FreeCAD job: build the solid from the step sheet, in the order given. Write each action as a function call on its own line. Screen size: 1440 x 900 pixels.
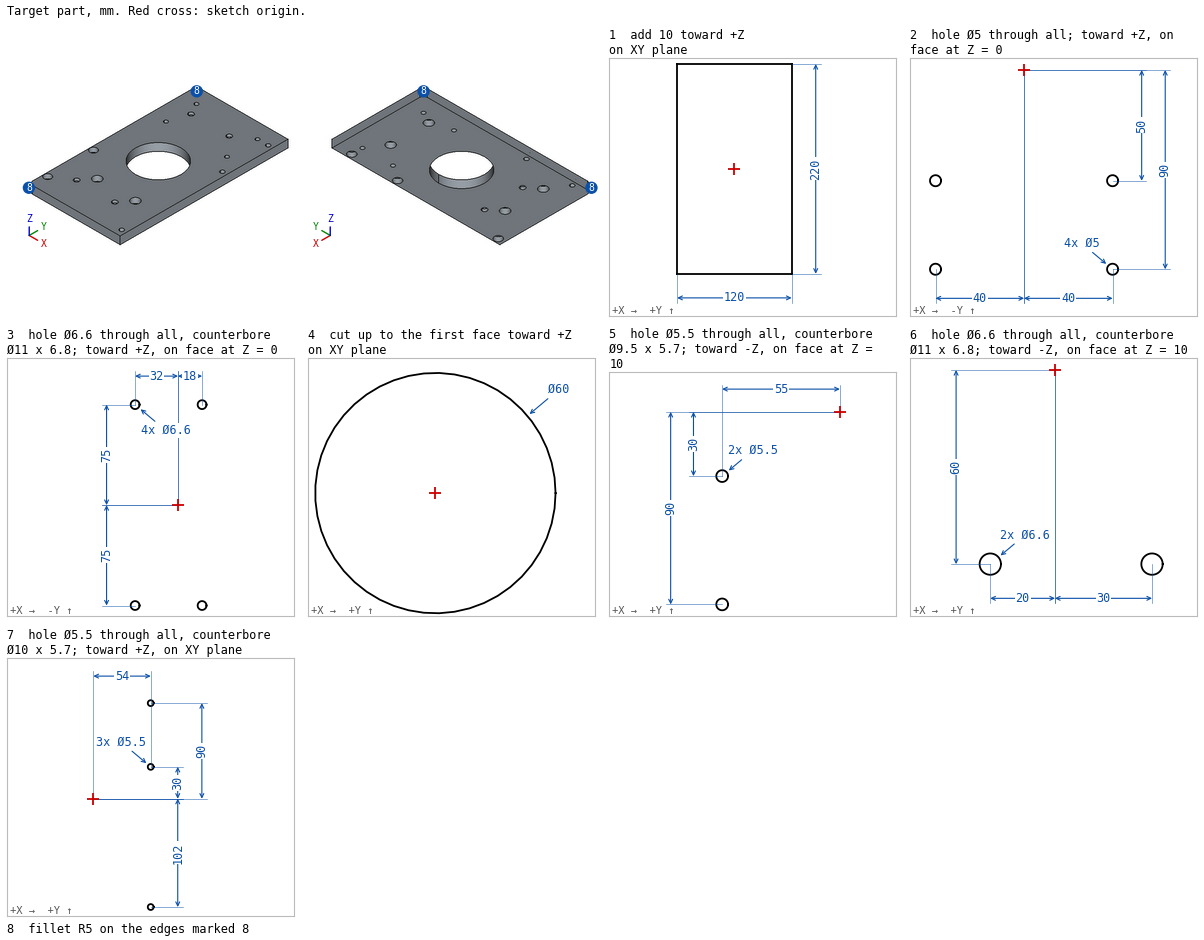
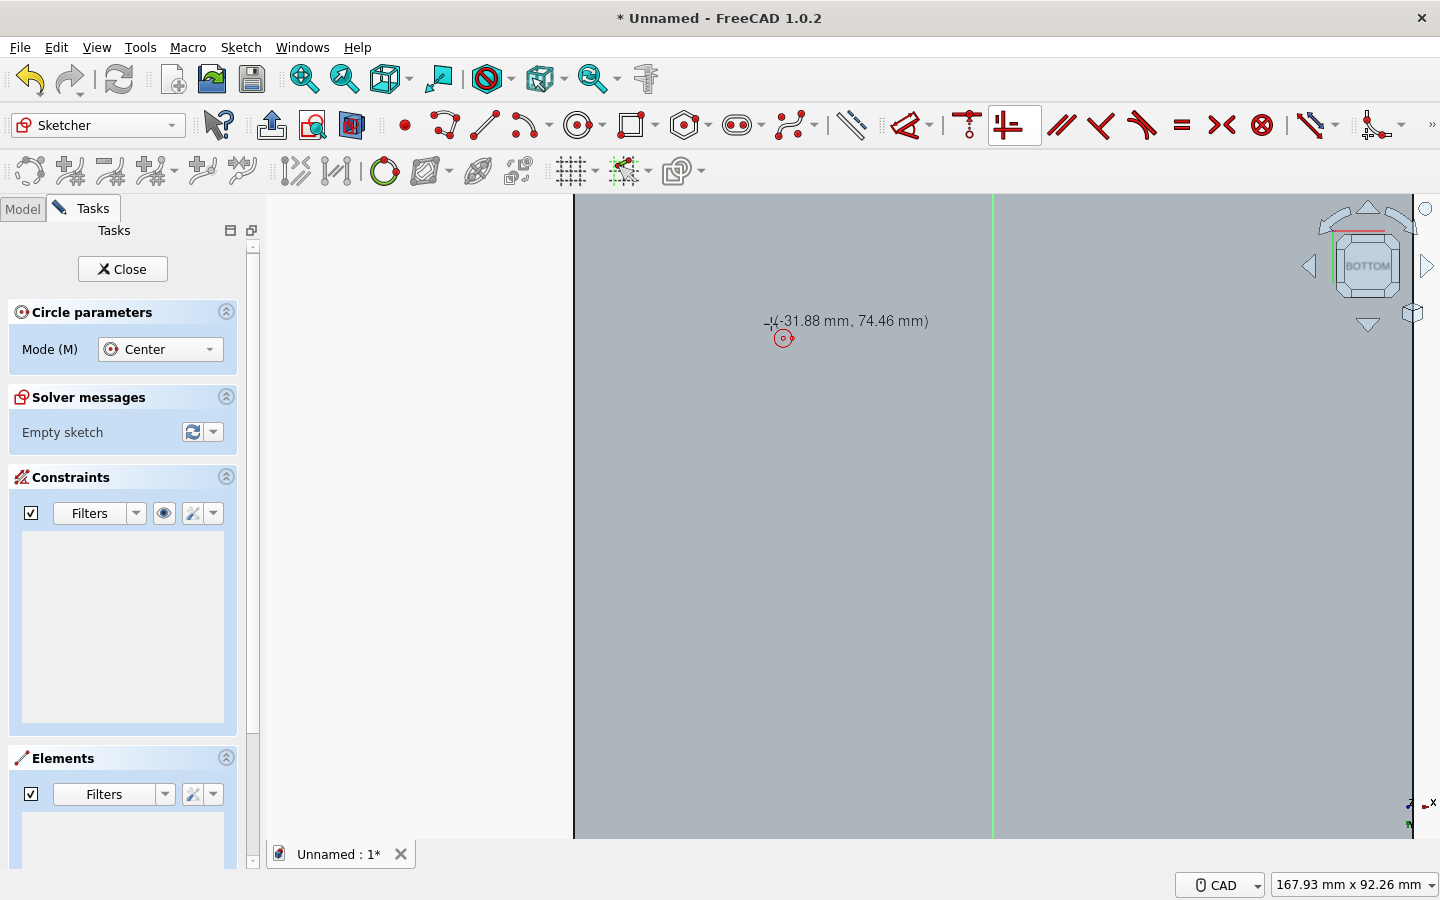
click(769, 323)
move(786, 306)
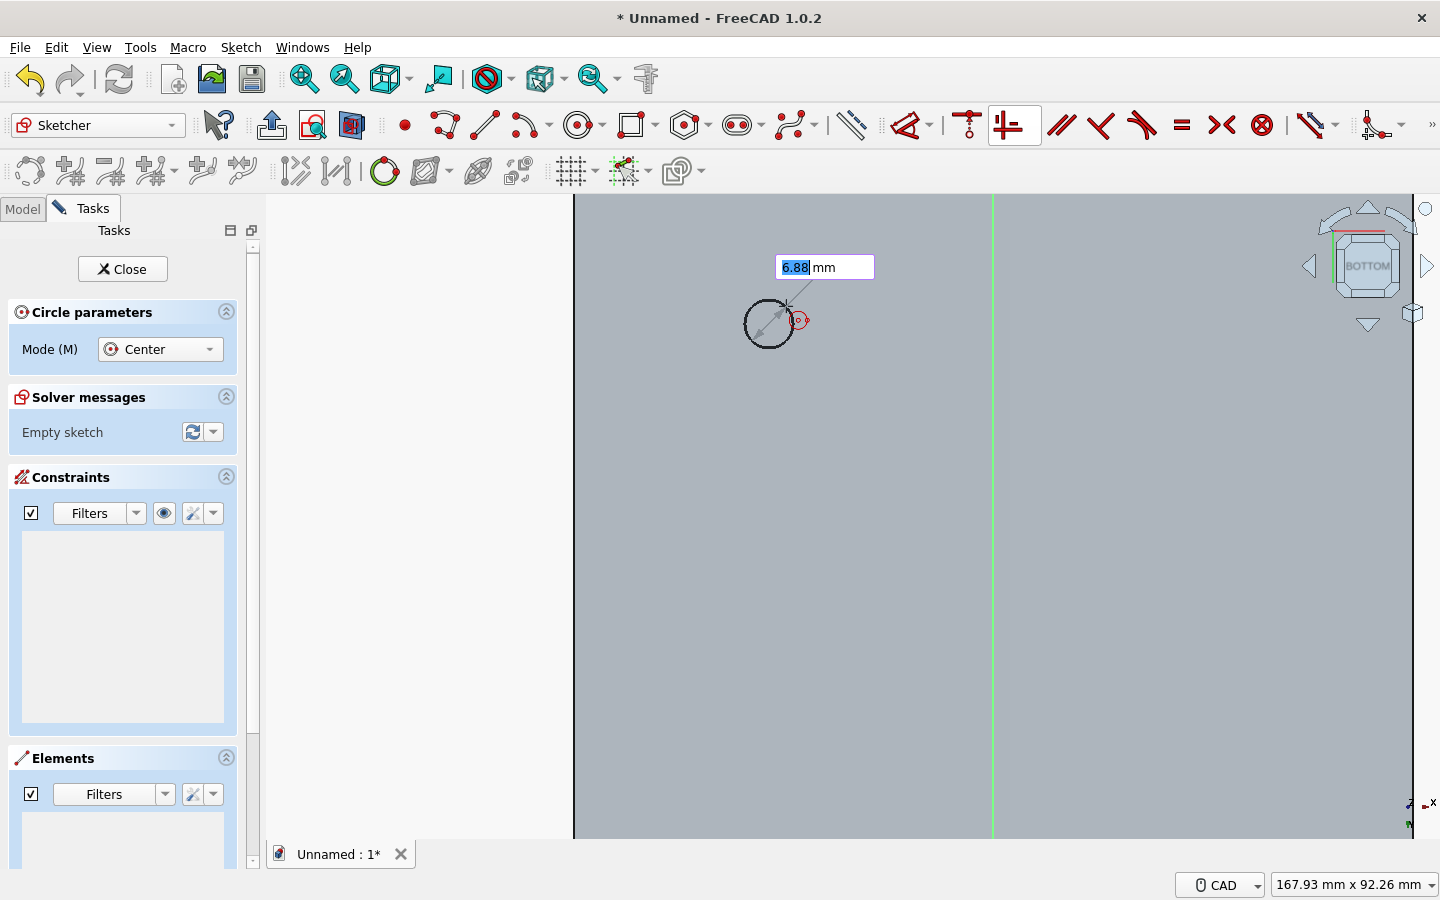
text(6.6)
key(Return)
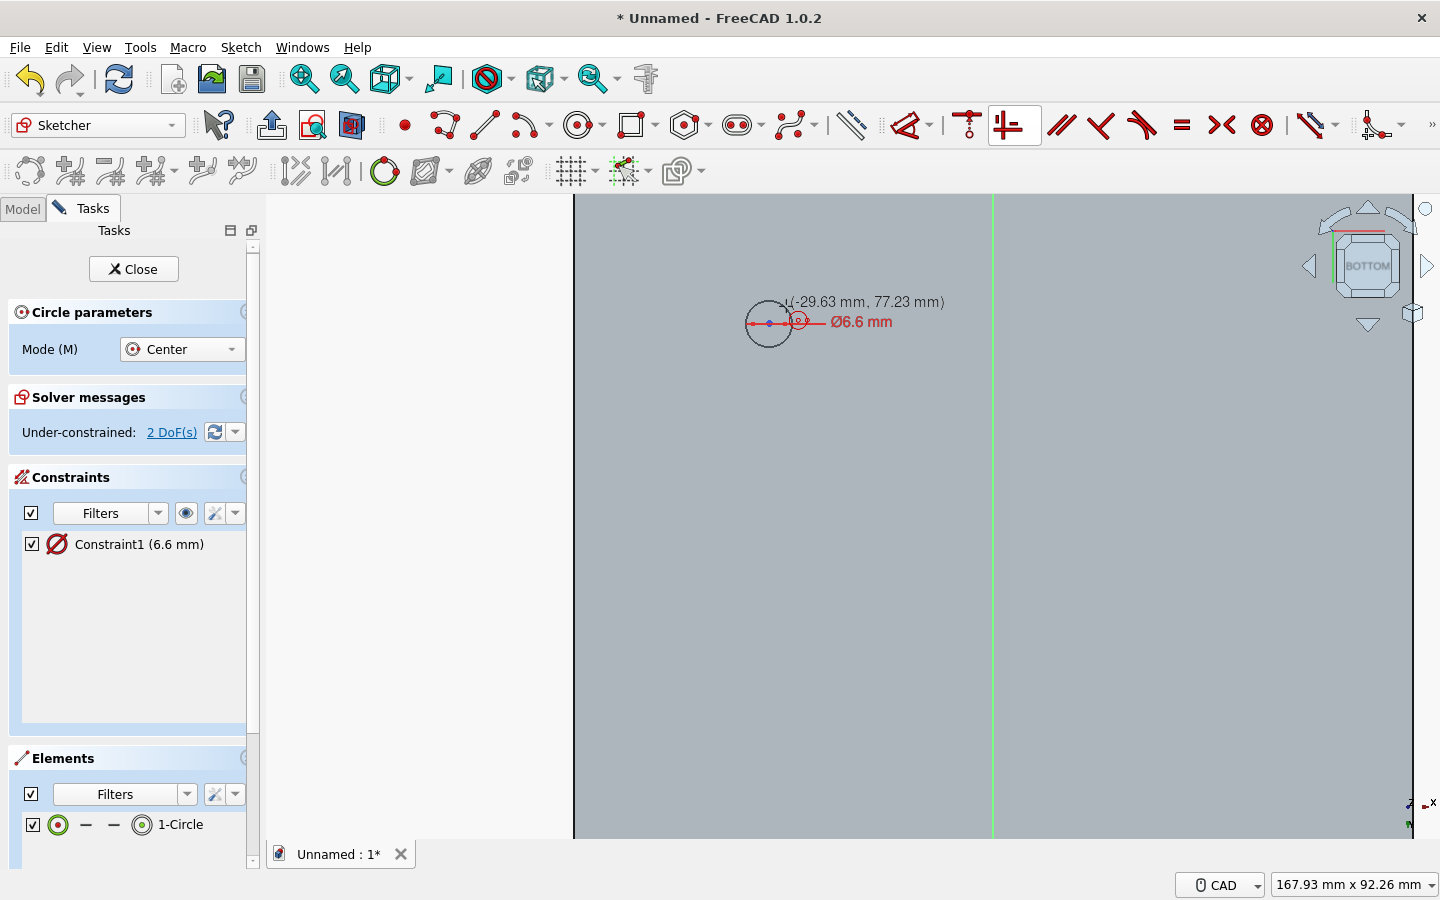
click(1119, 323)
move(1135, 306)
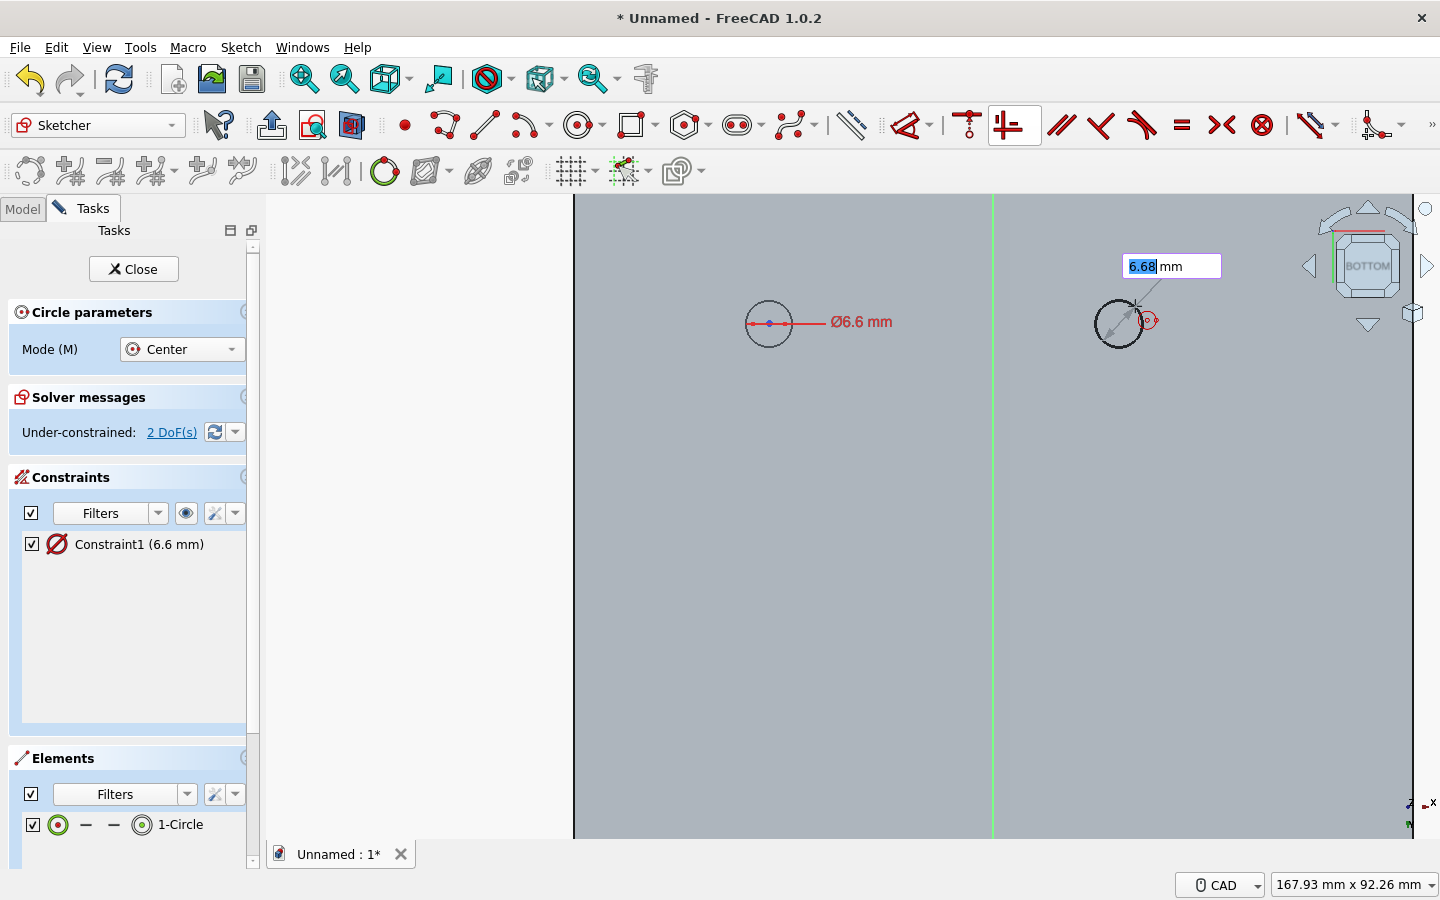
text(6.6)
key(Return)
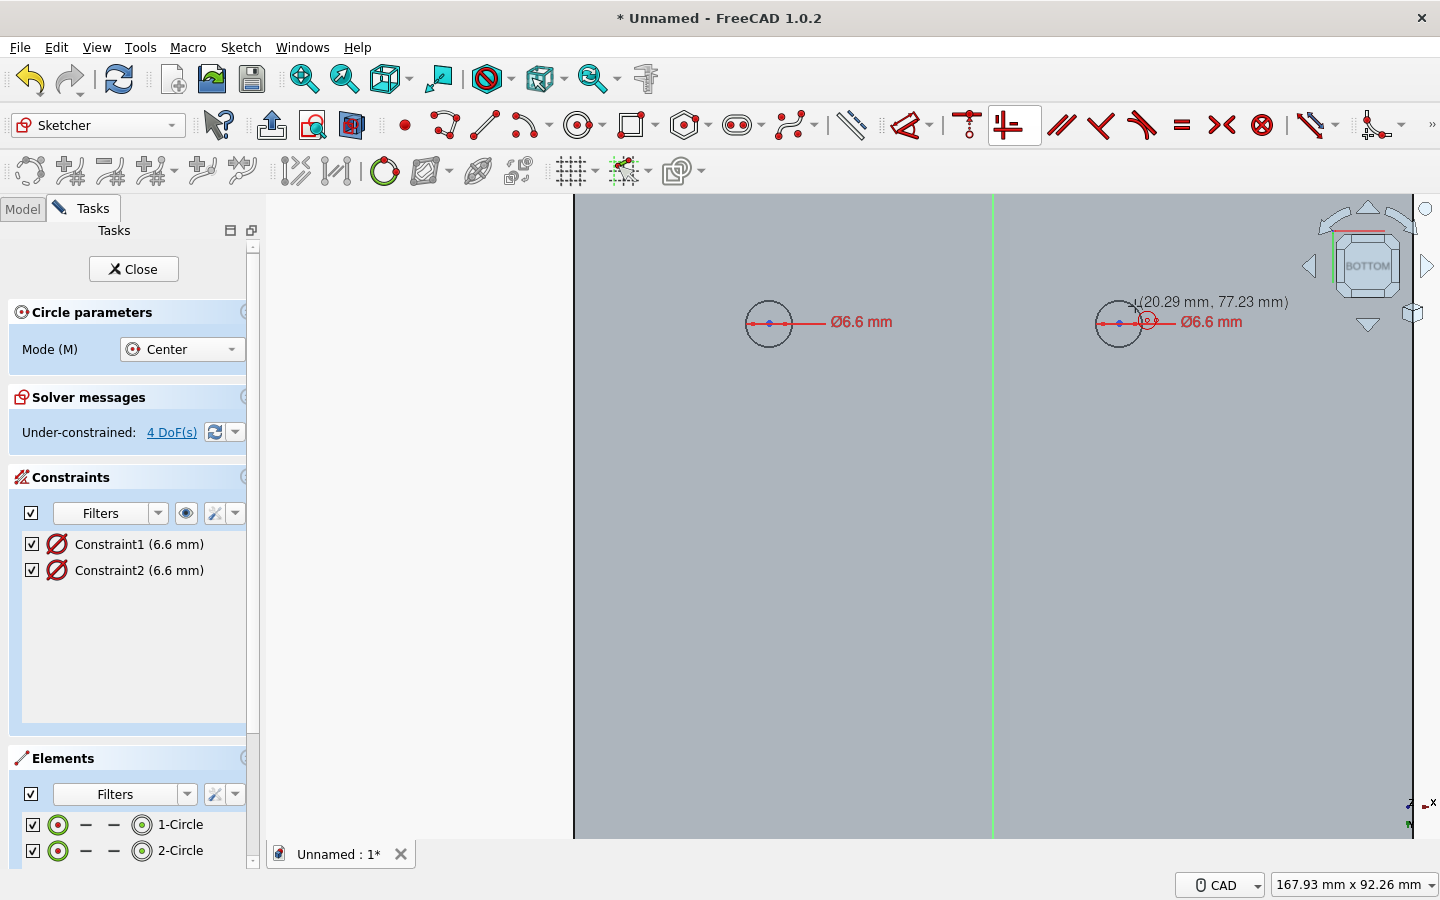
scroll(692, 324, down, 5)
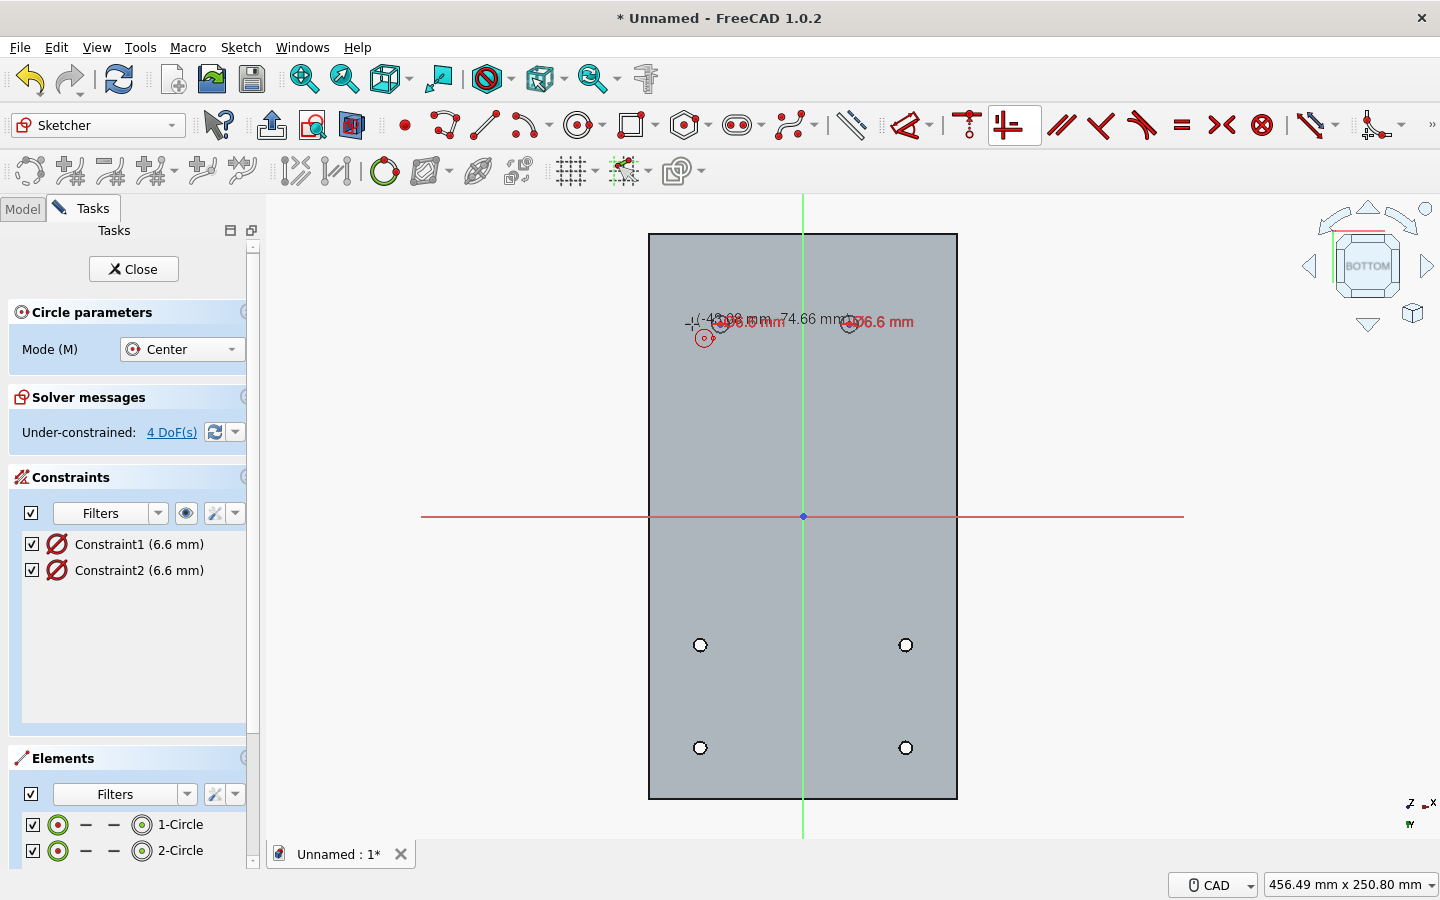
scroll(721, 709, up, 5)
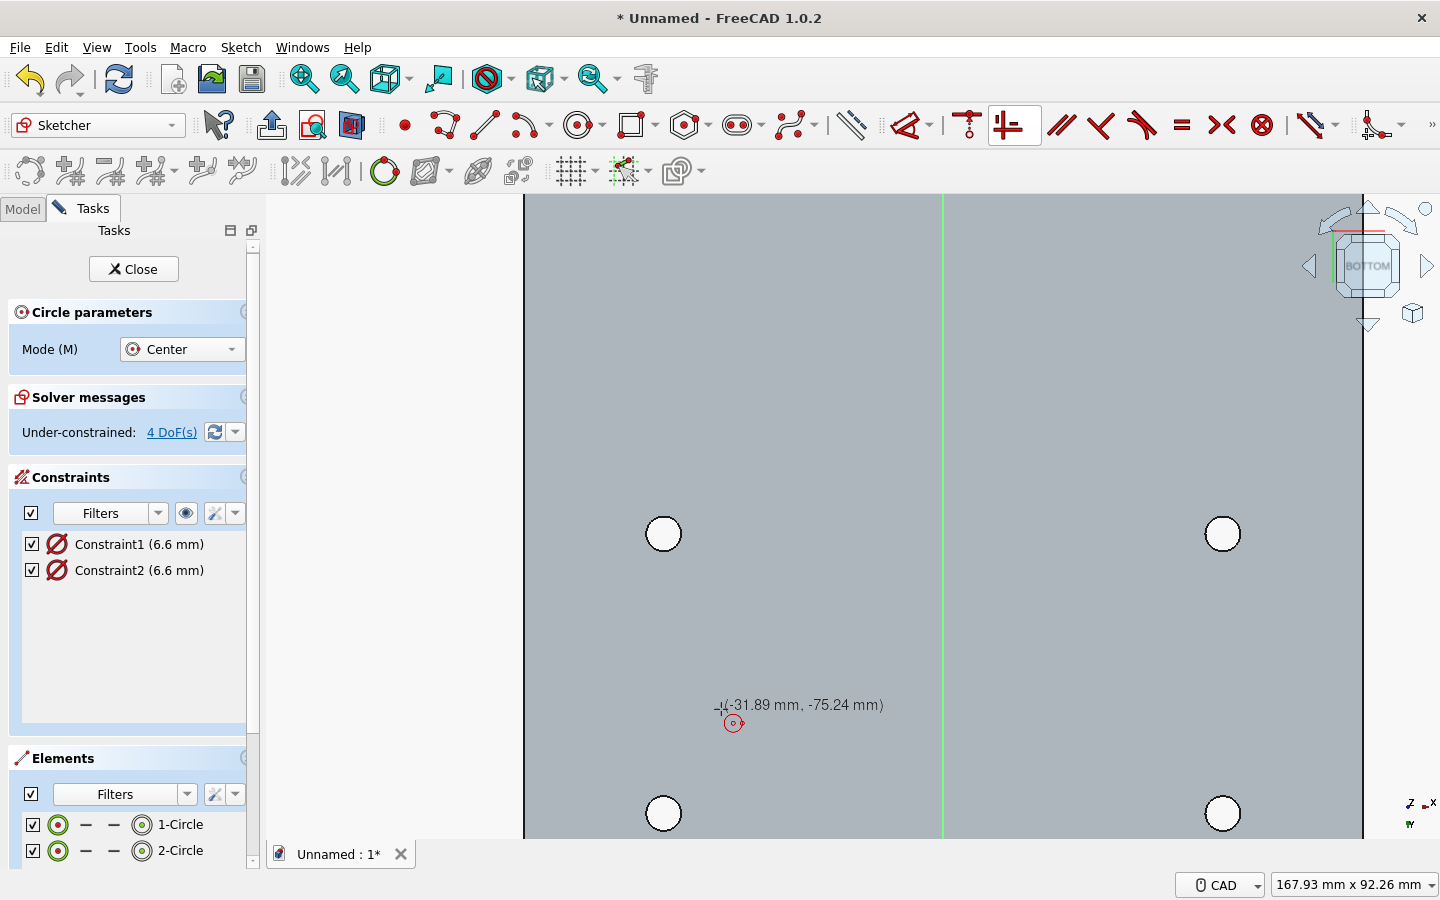
click(720, 709)
move(736, 692)